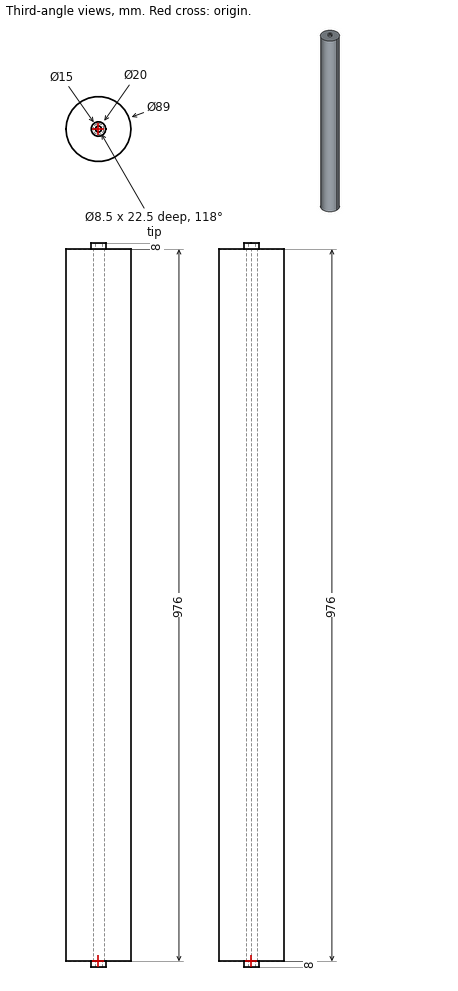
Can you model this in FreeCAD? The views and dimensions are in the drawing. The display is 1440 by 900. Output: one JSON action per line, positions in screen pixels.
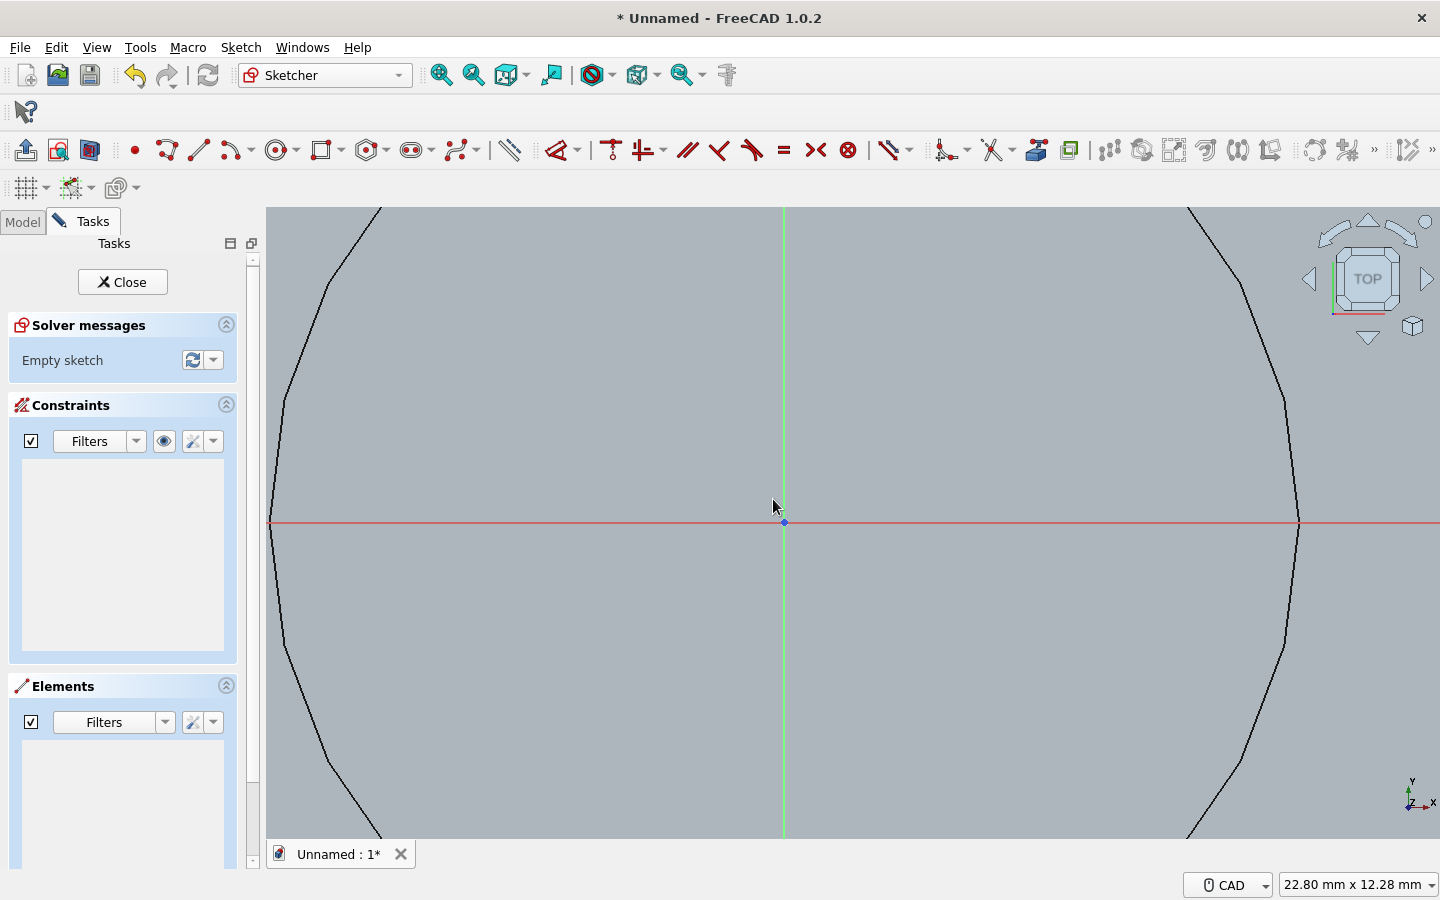
{"action": "left_click", "coordinate": [276, 150]}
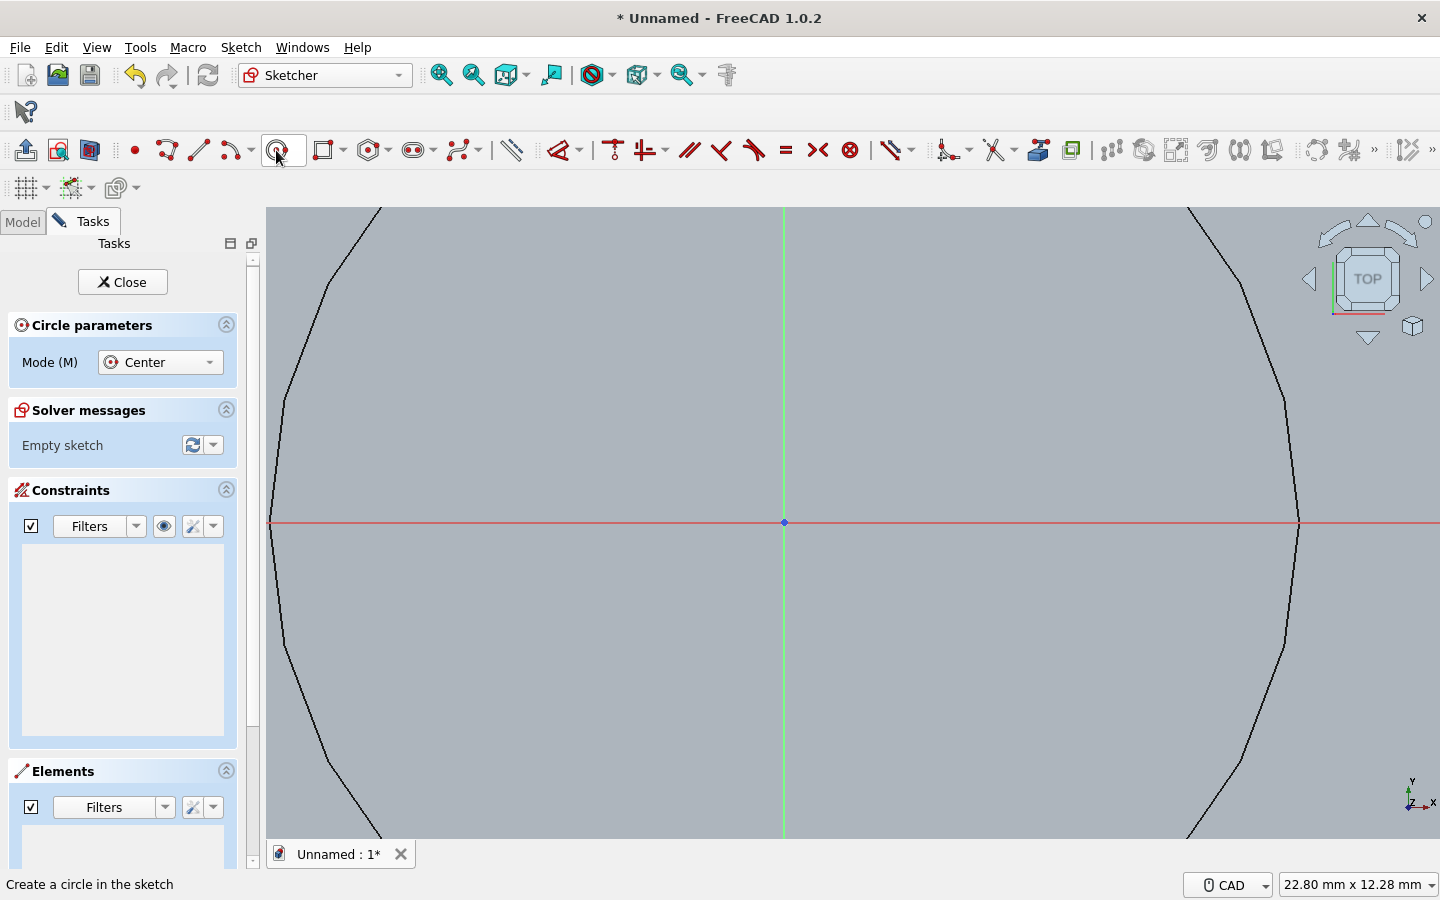
{"action": "left_click", "coordinate": [784, 523]}
{"action": "left_click", "coordinate": [939, 368]}
{"action": "key", "text": "Escape"}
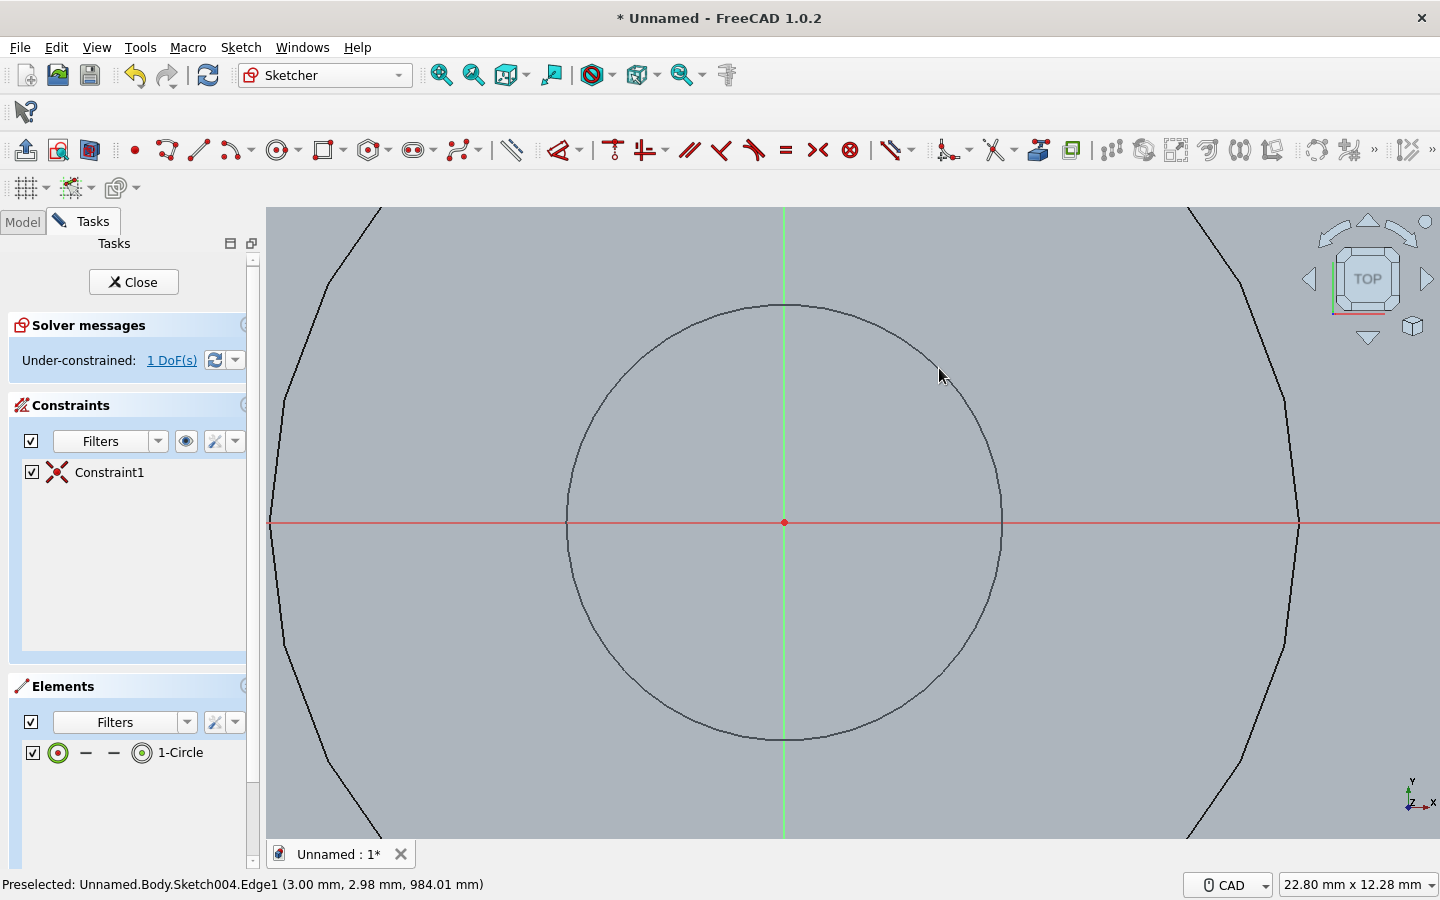
{"action": "left_click", "coordinate": [558, 150]}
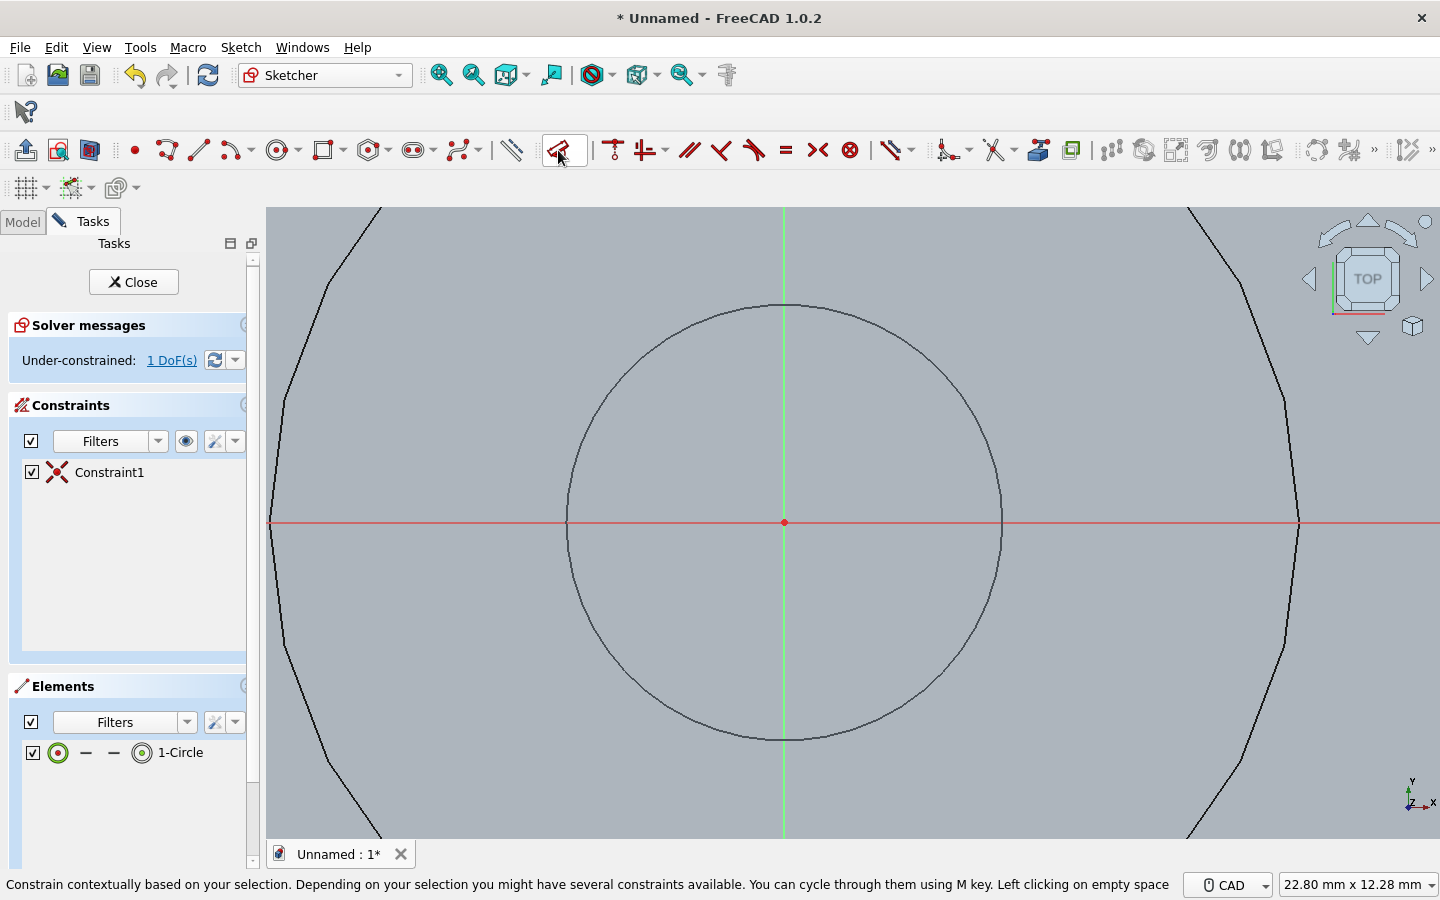
{"action": "left_click", "coordinate": [938, 368]}
{"action": "left_click", "coordinate": [961, 345]}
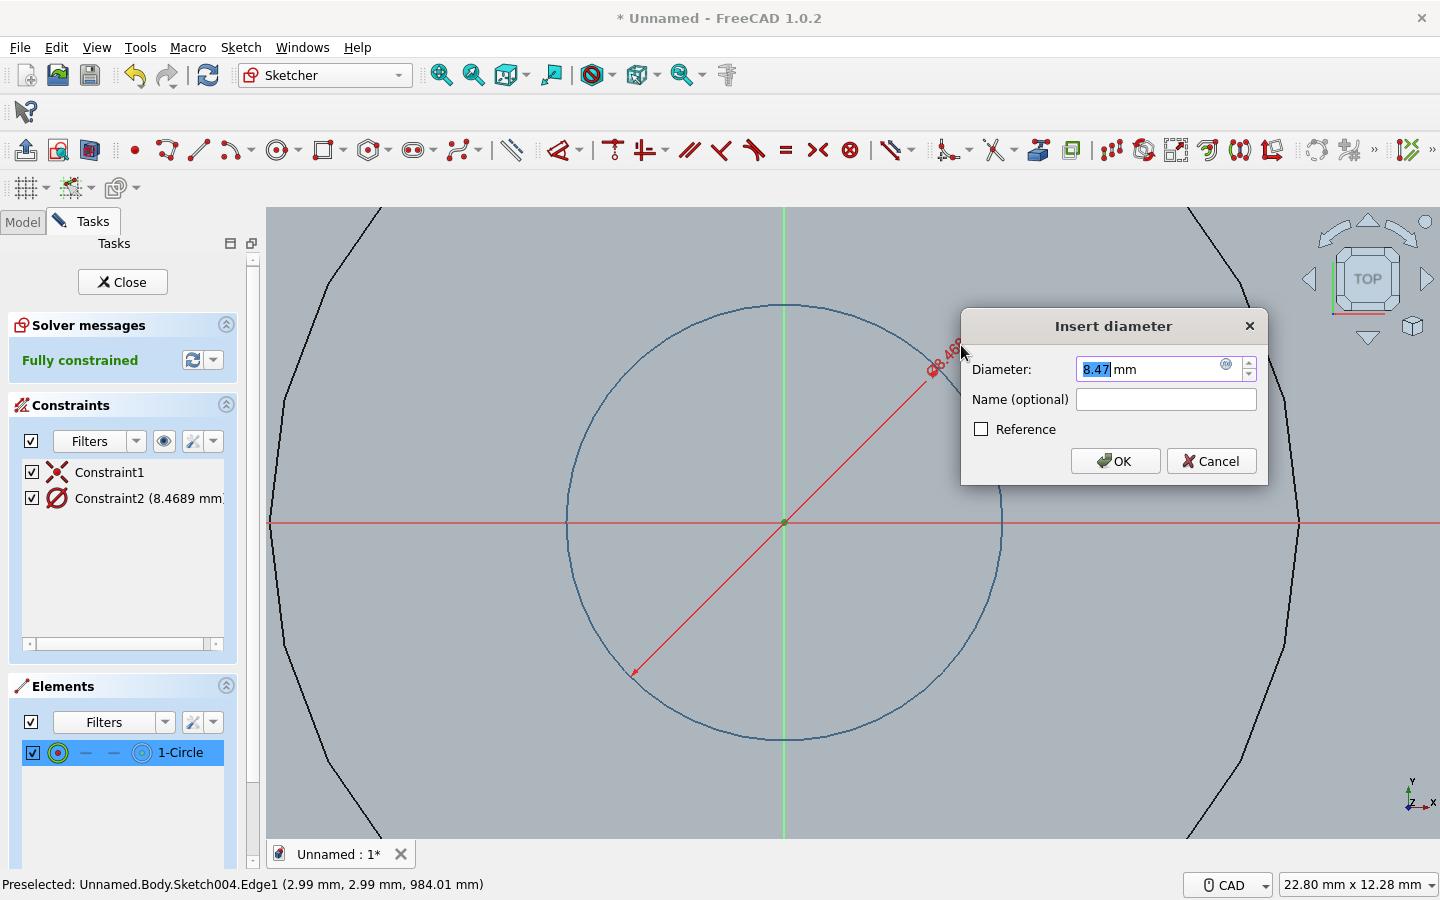
{"action": "type", "text": "8.5"}
{"action": "key", "text": "Return"}
{"action": "key", "text": "Escape"}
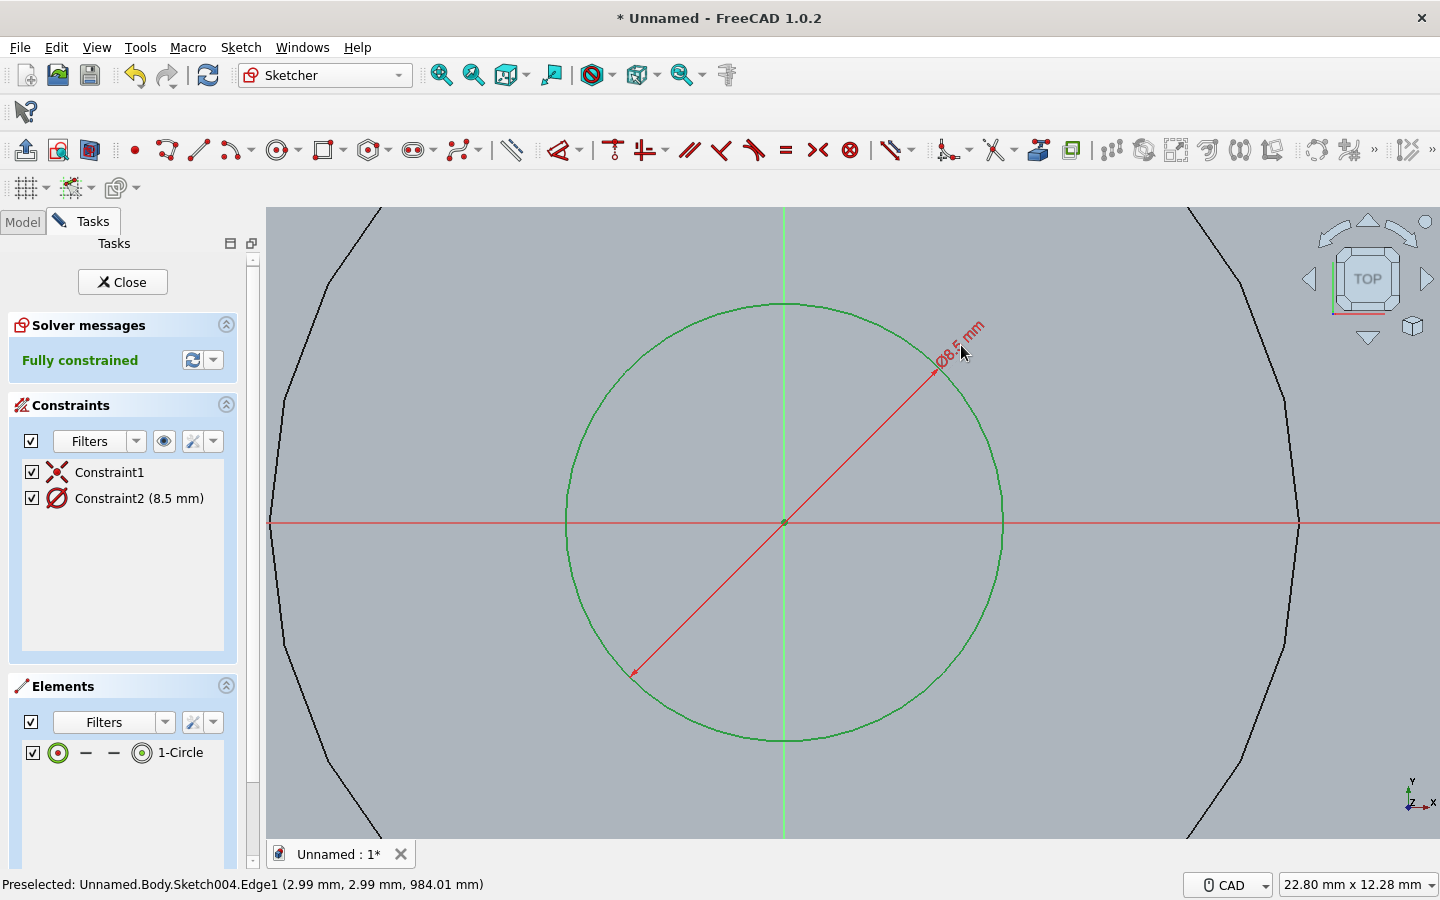
{"action": "left_click", "coordinate": [123, 282]}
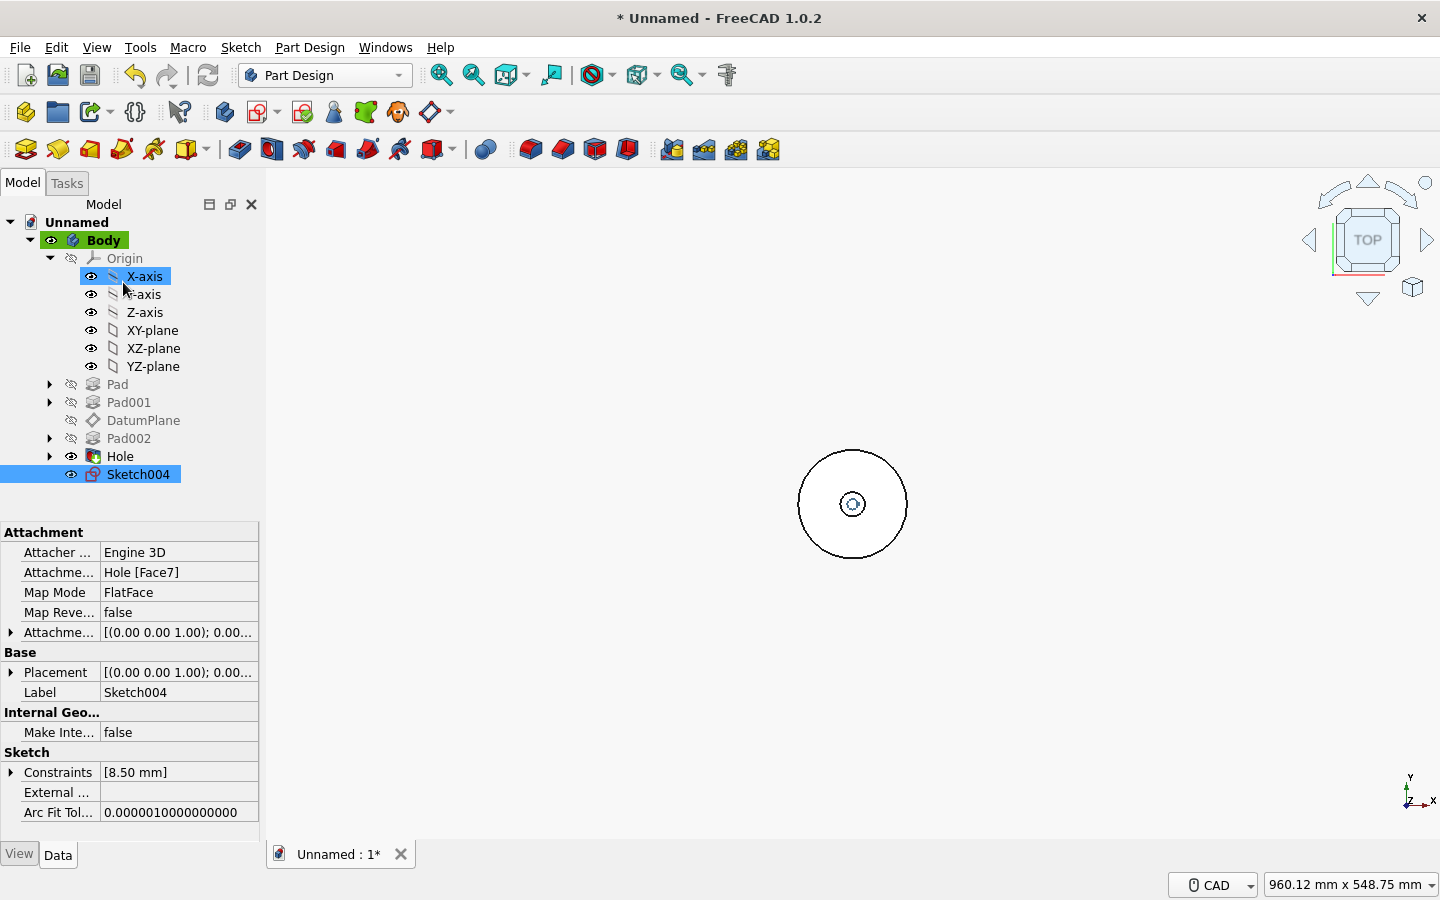
{"action": "left_click", "coordinate": [272, 150]}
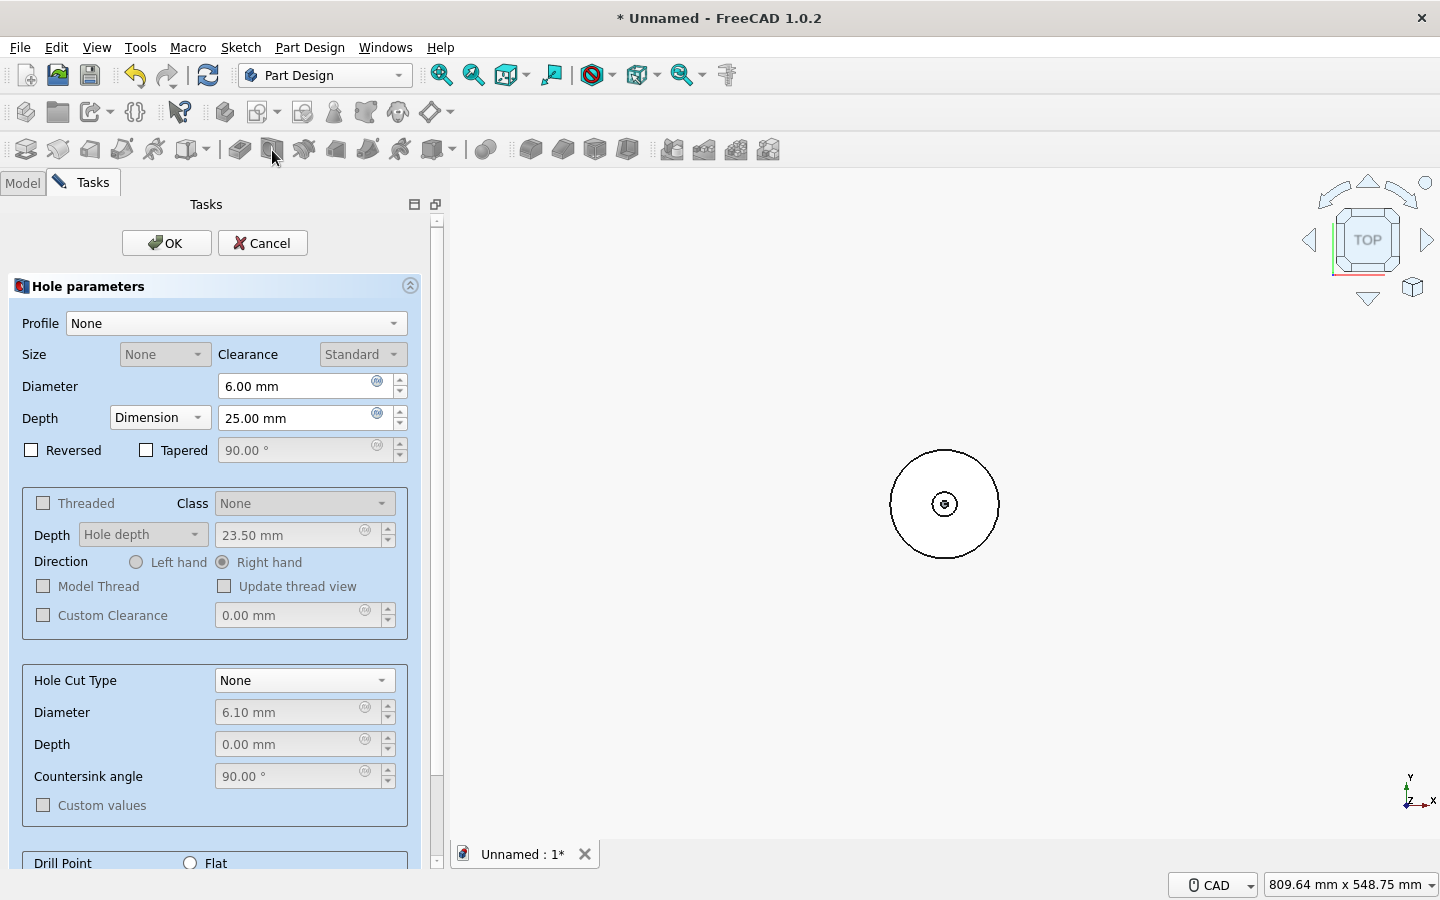
{"action": "triple_click", "coordinate": [305, 386]}